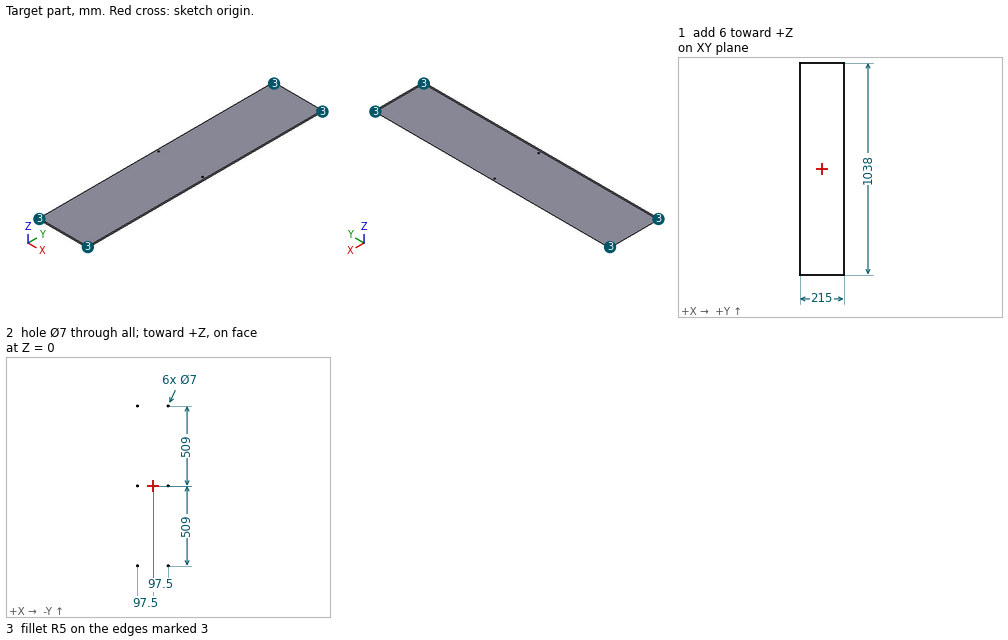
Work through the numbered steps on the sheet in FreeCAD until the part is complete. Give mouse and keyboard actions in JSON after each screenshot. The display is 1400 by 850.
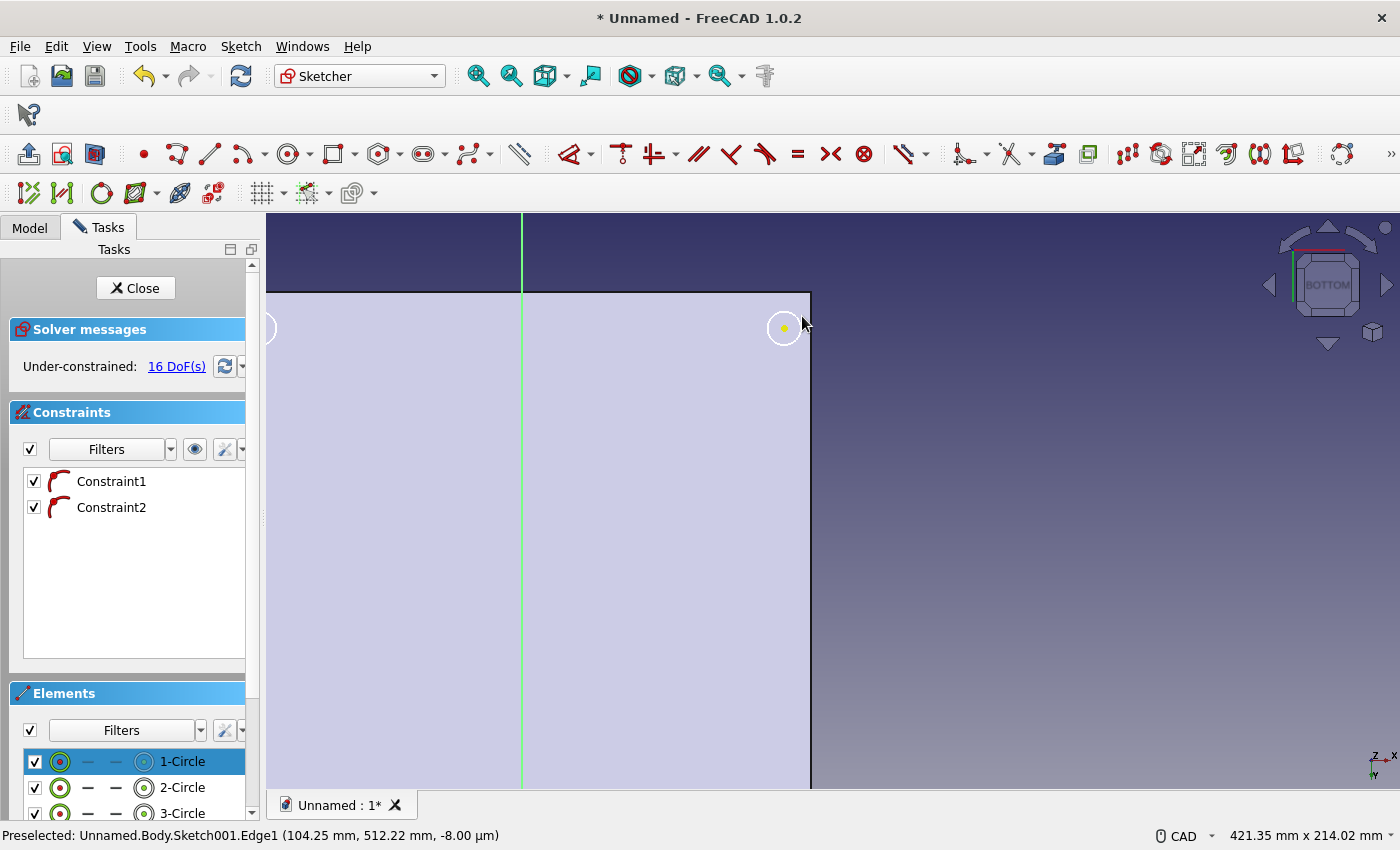
{"action": "left_click", "coordinate": [796, 317]}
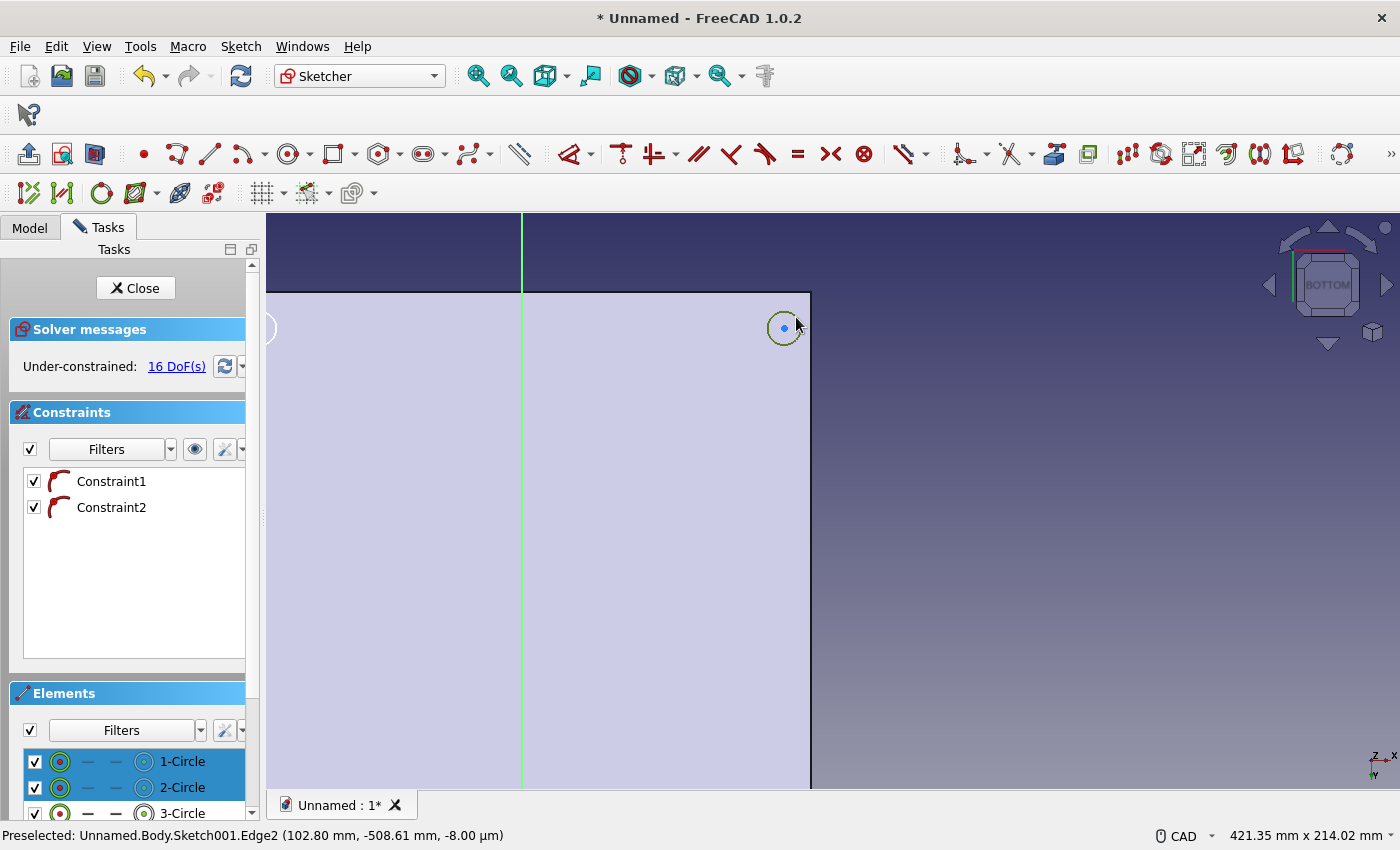
{"action": "scroll", "coordinate": [802, 315], "scroll_direction": "down", "scroll_amount": 10}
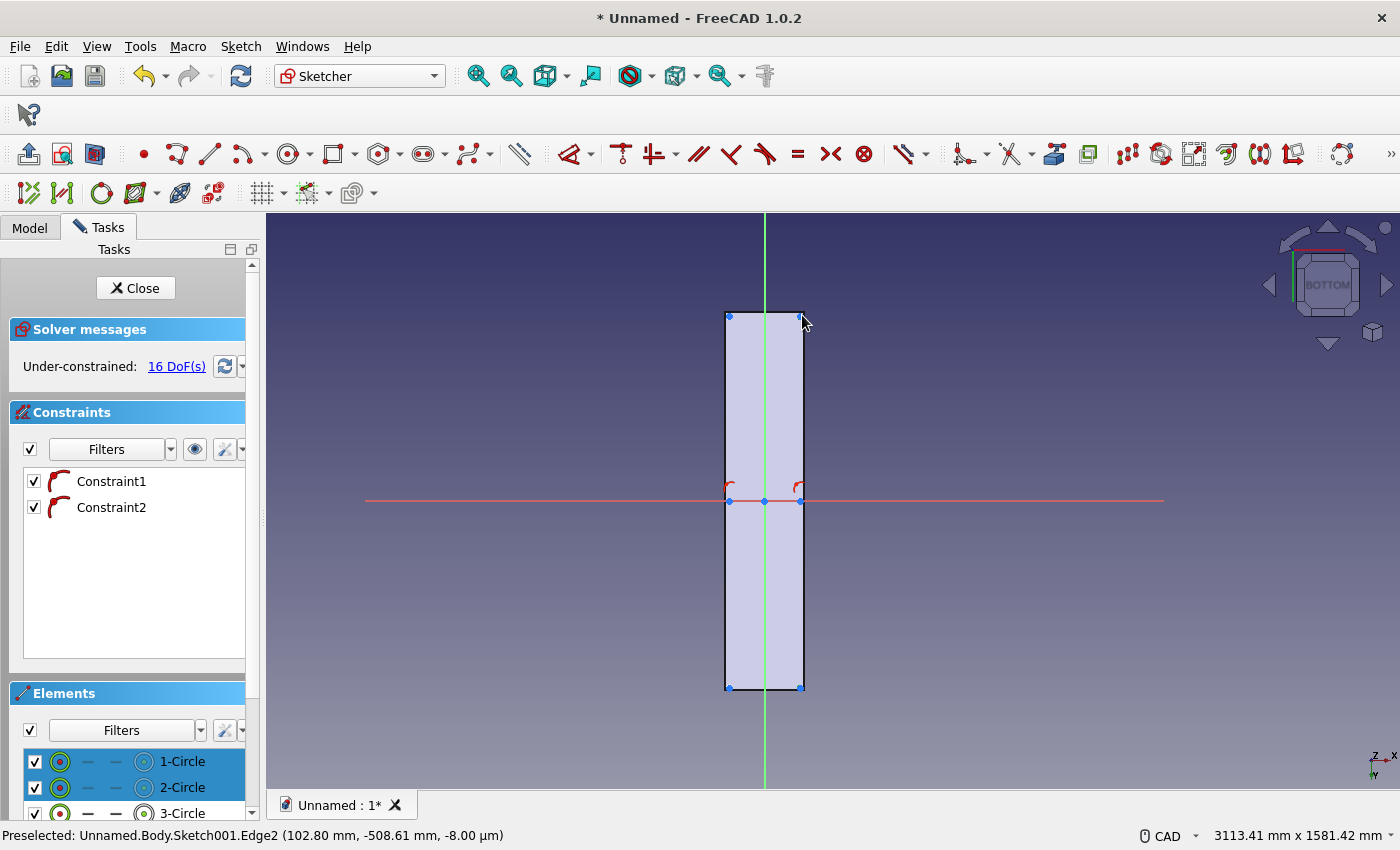
{"action": "scroll", "coordinate": [731, 686], "scroll_direction": "up", "scroll_amount": 9}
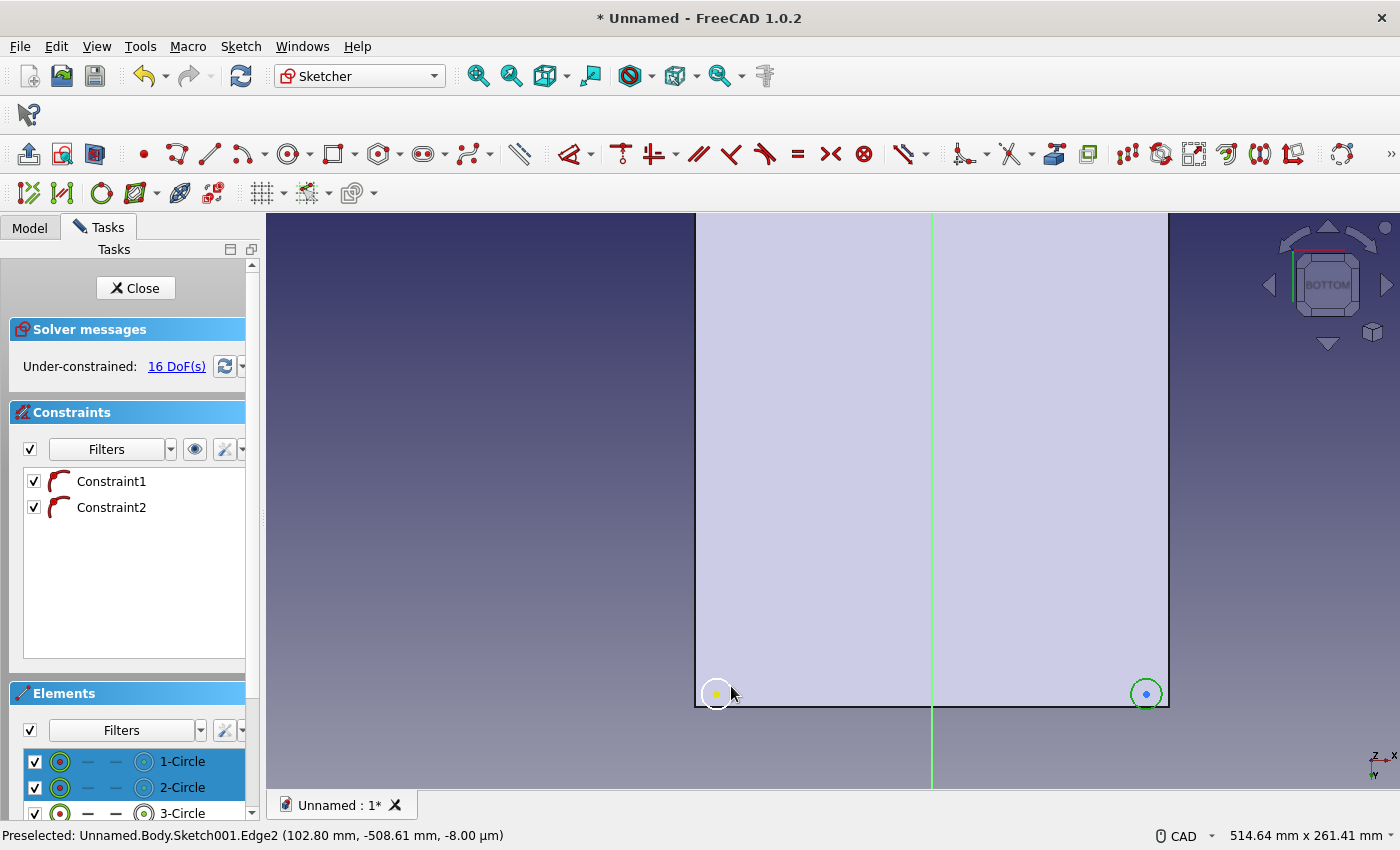
{"action": "left_click", "coordinate": [728, 683]}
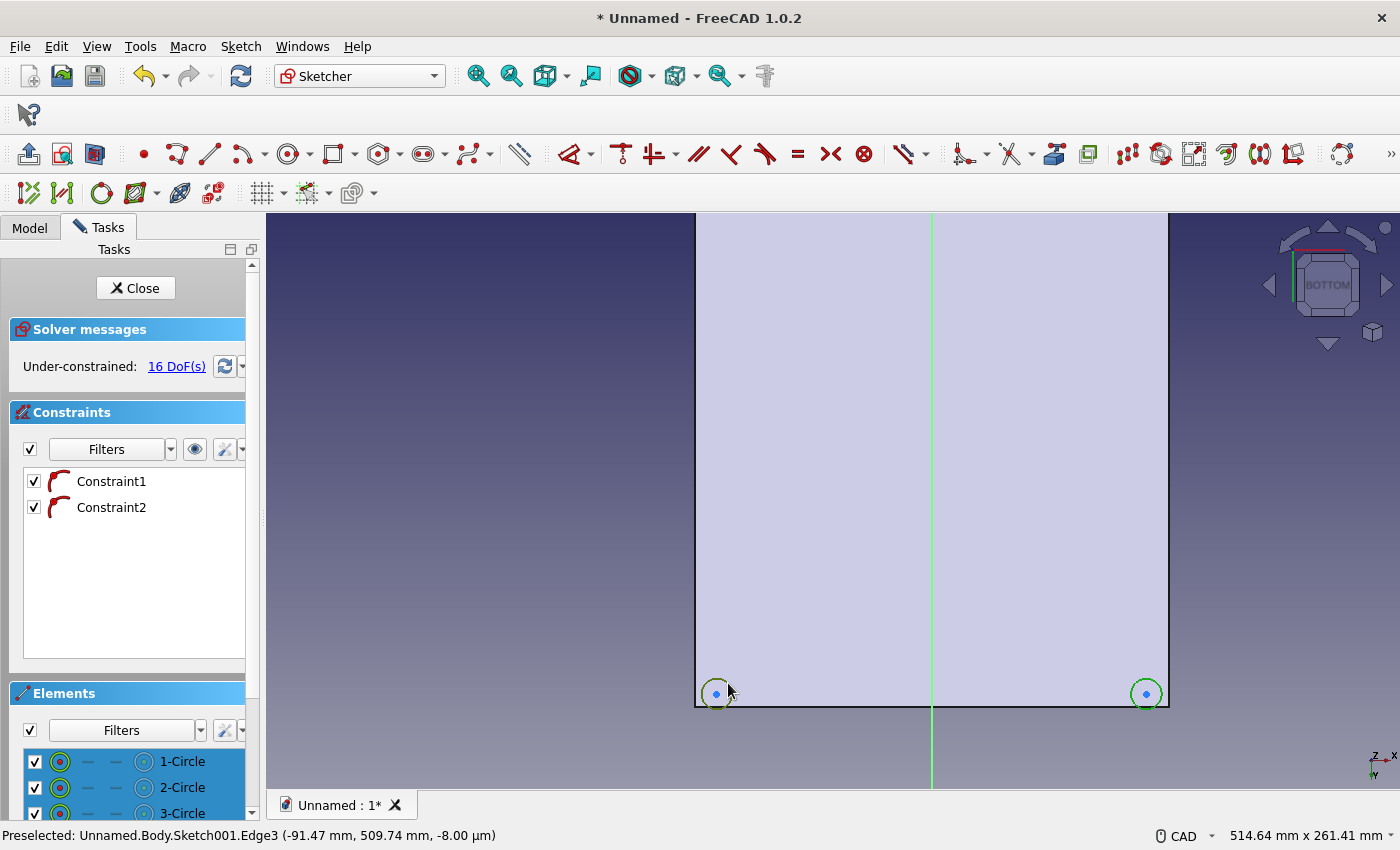
{"action": "scroll", "coordinate": [731, 687], "scroll_direction": "down", "scroll_amount": 9}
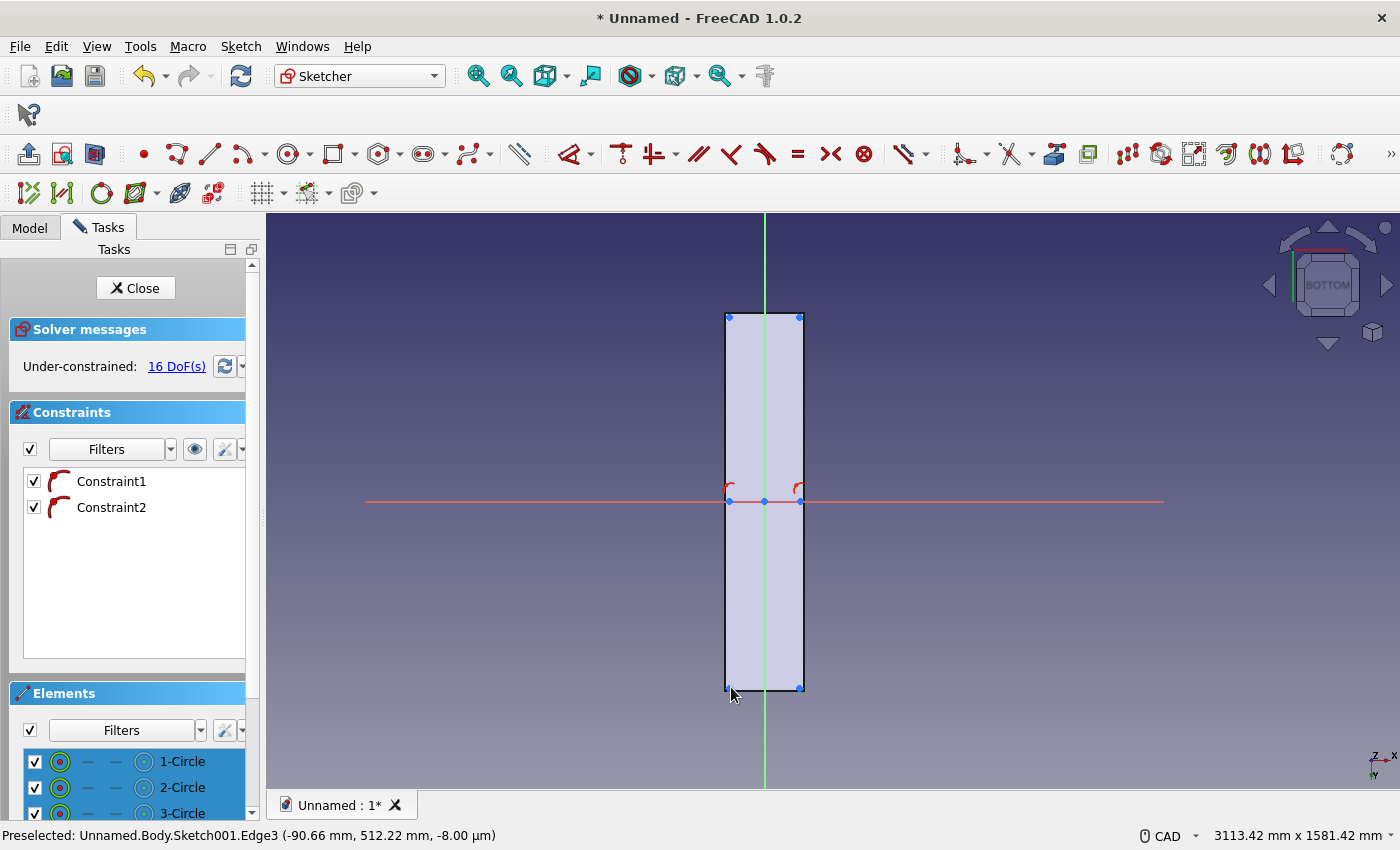
{"action": "scroll", "coordinate": [731, 316], "scroll_direction": "up", "scroll_amount": 10}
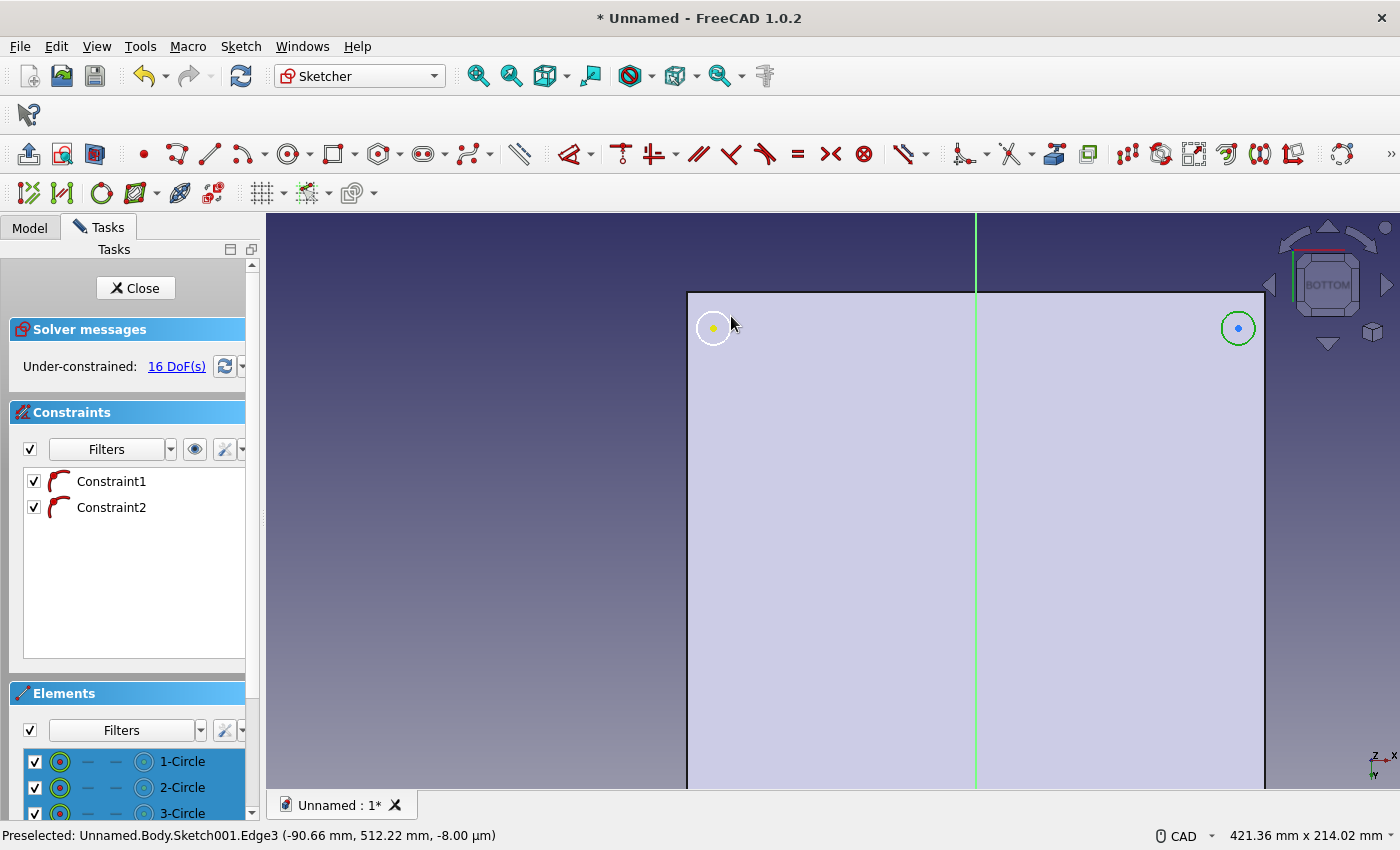
{"action": "left_click", "coordinate": [725, 316]}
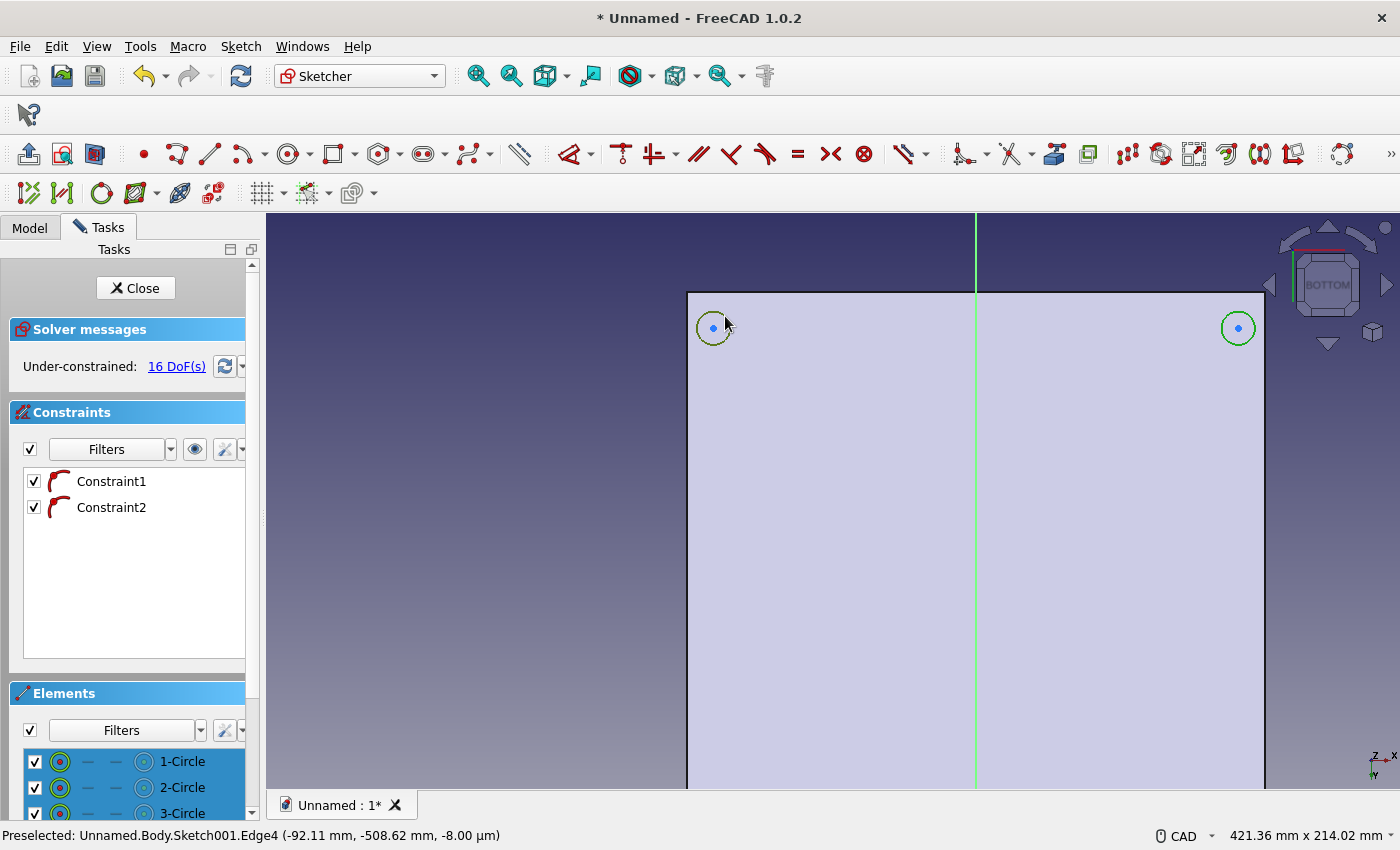
{"action": "scroll", "coordinate": [731, 315], "scroll_direction": "down", "scroll_amount": 10}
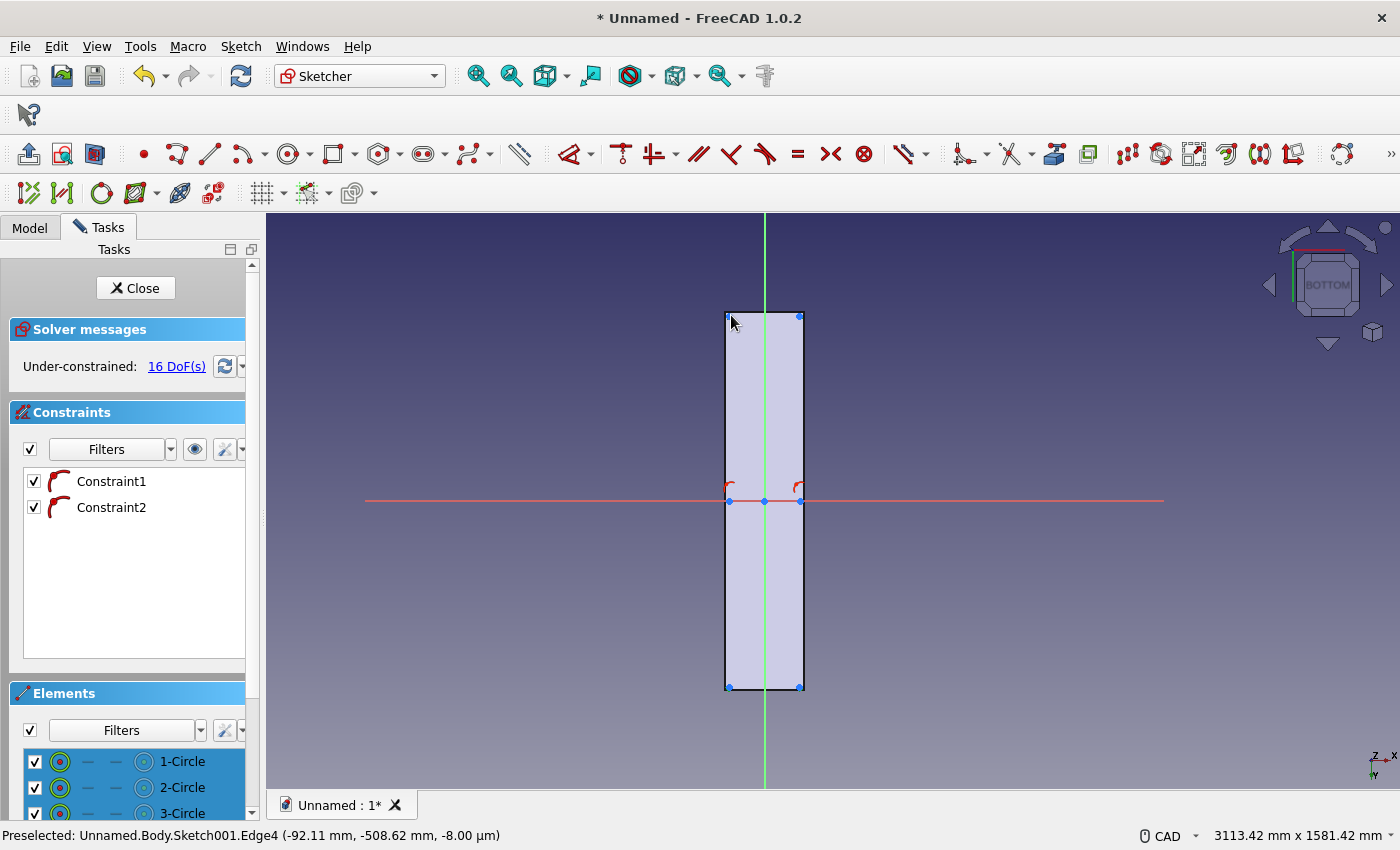
{"action": "scroll", "coordinate": [800, 500], "scroll_direction": "up", "scroll_amount": 12}